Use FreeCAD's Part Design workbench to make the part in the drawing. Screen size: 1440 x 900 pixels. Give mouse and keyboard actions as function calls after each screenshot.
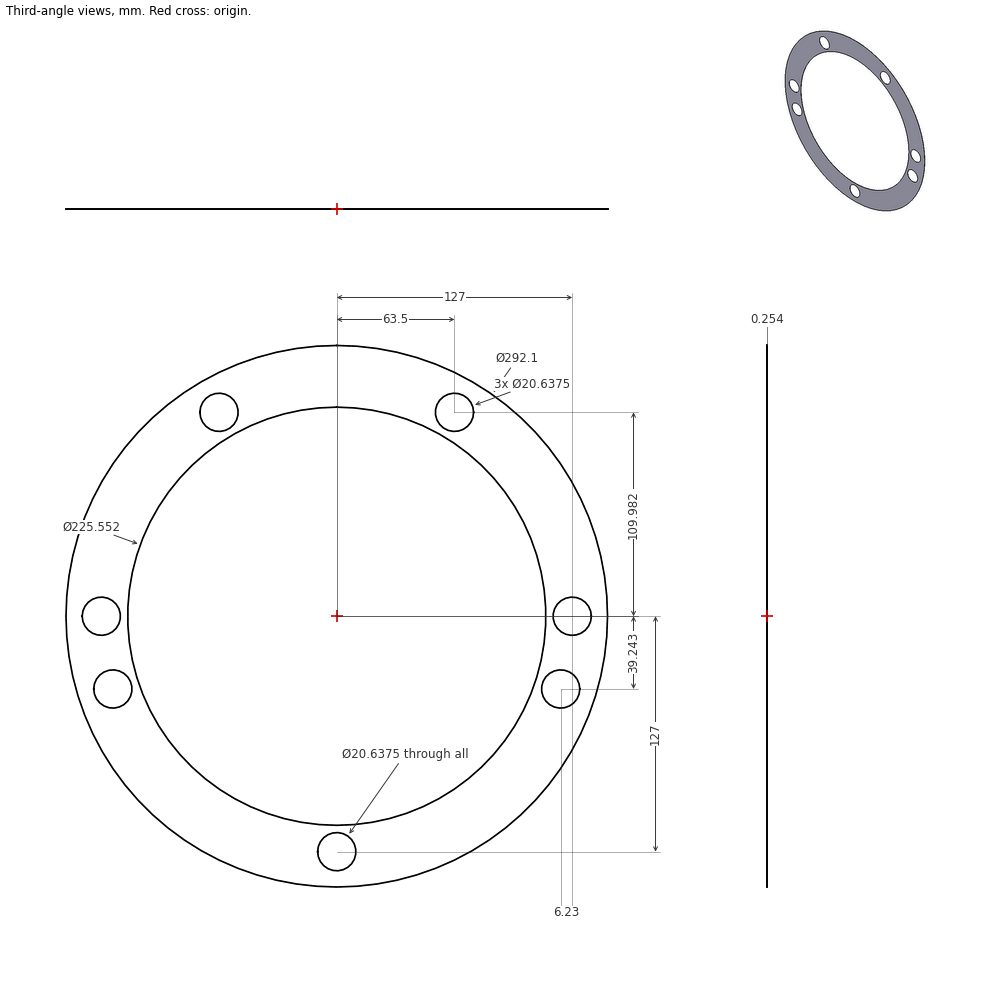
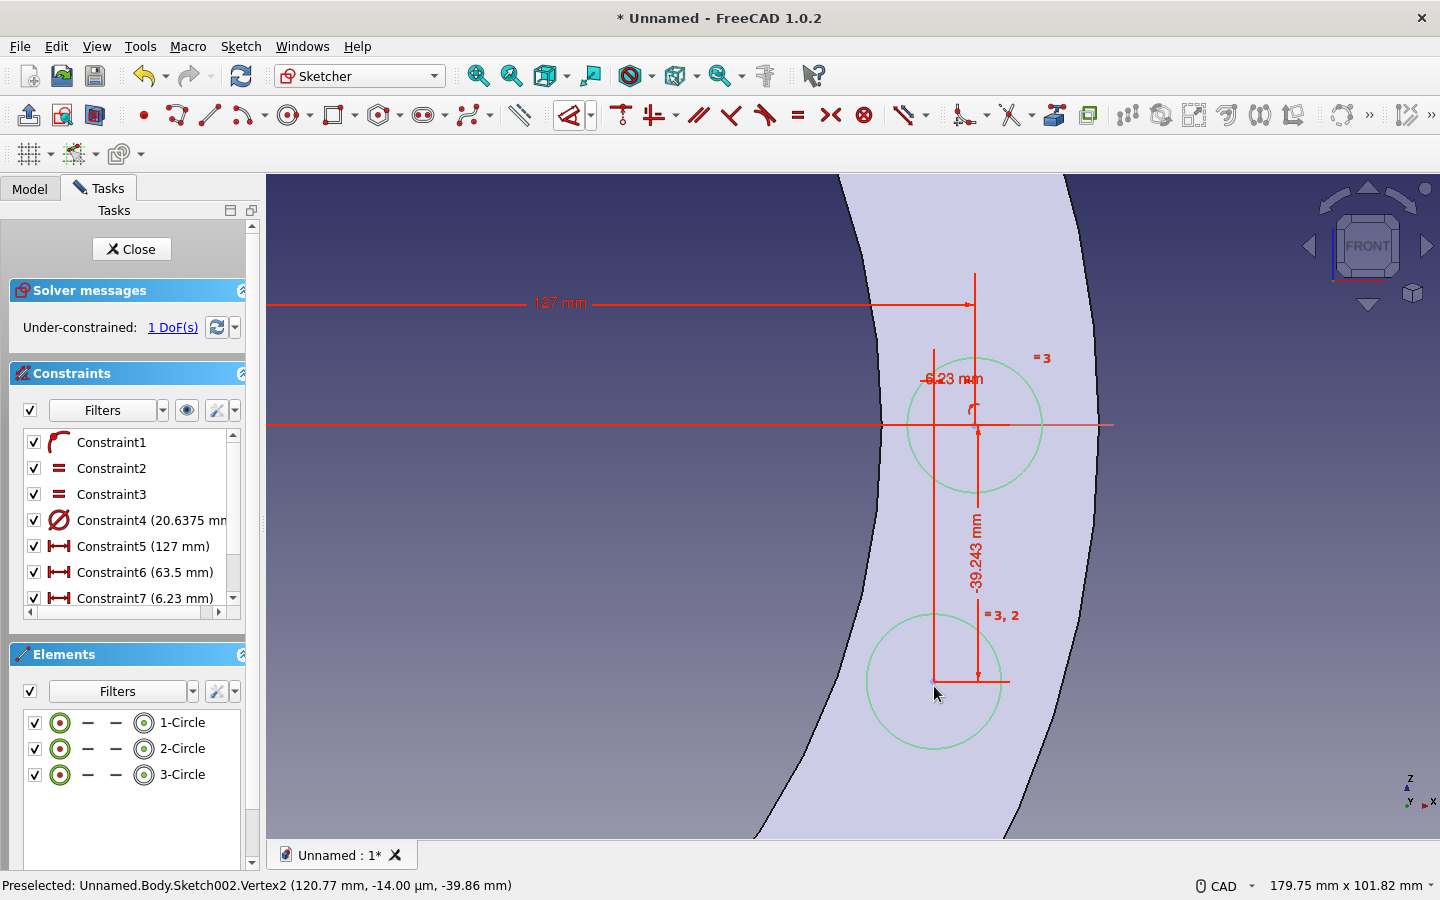
scroll(896, 688, down, 5)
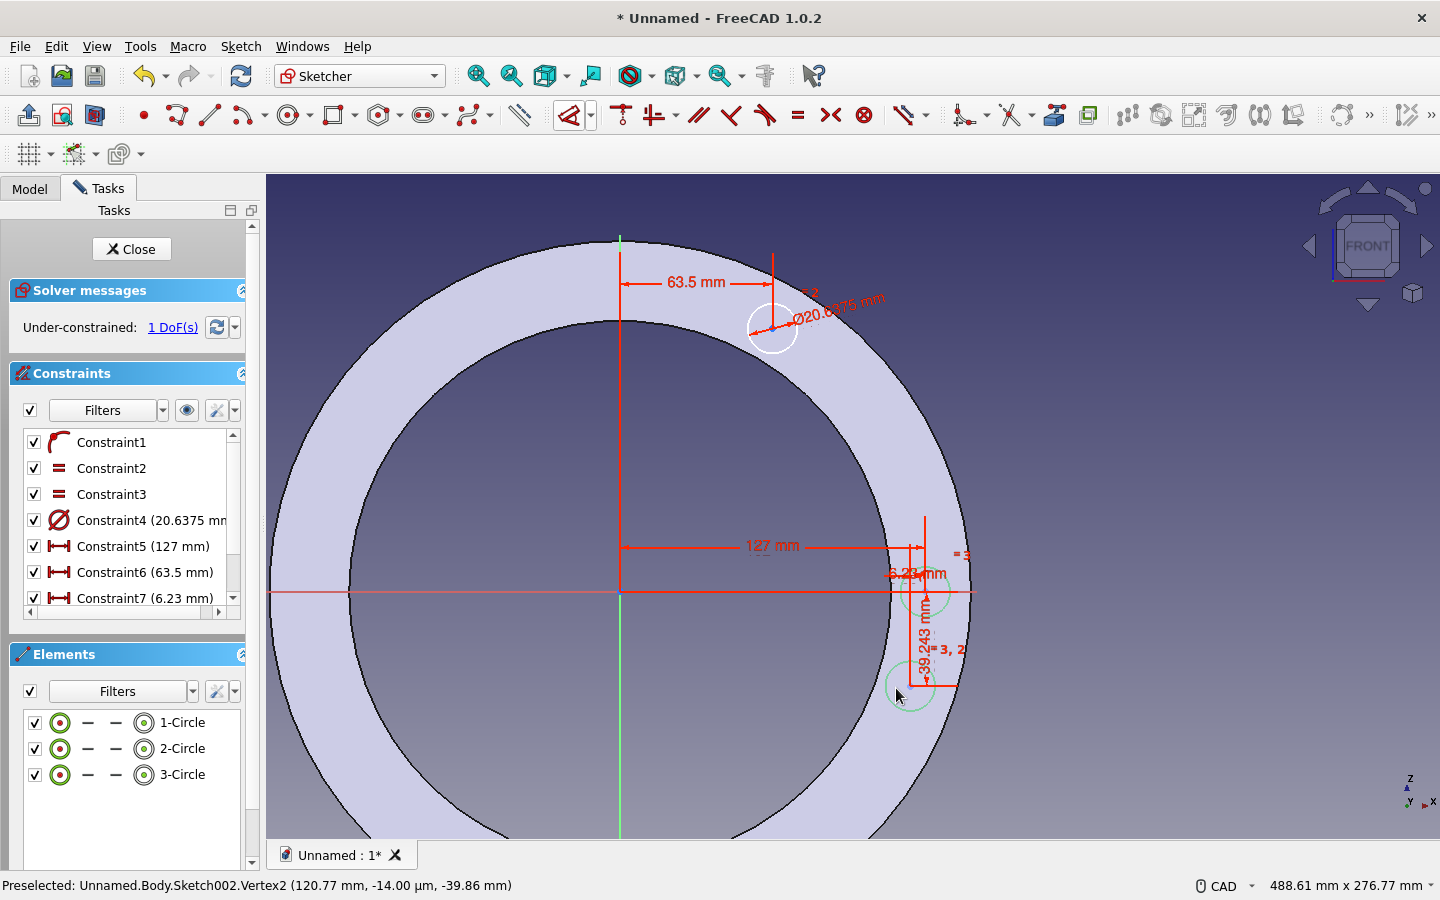
click(773, 329)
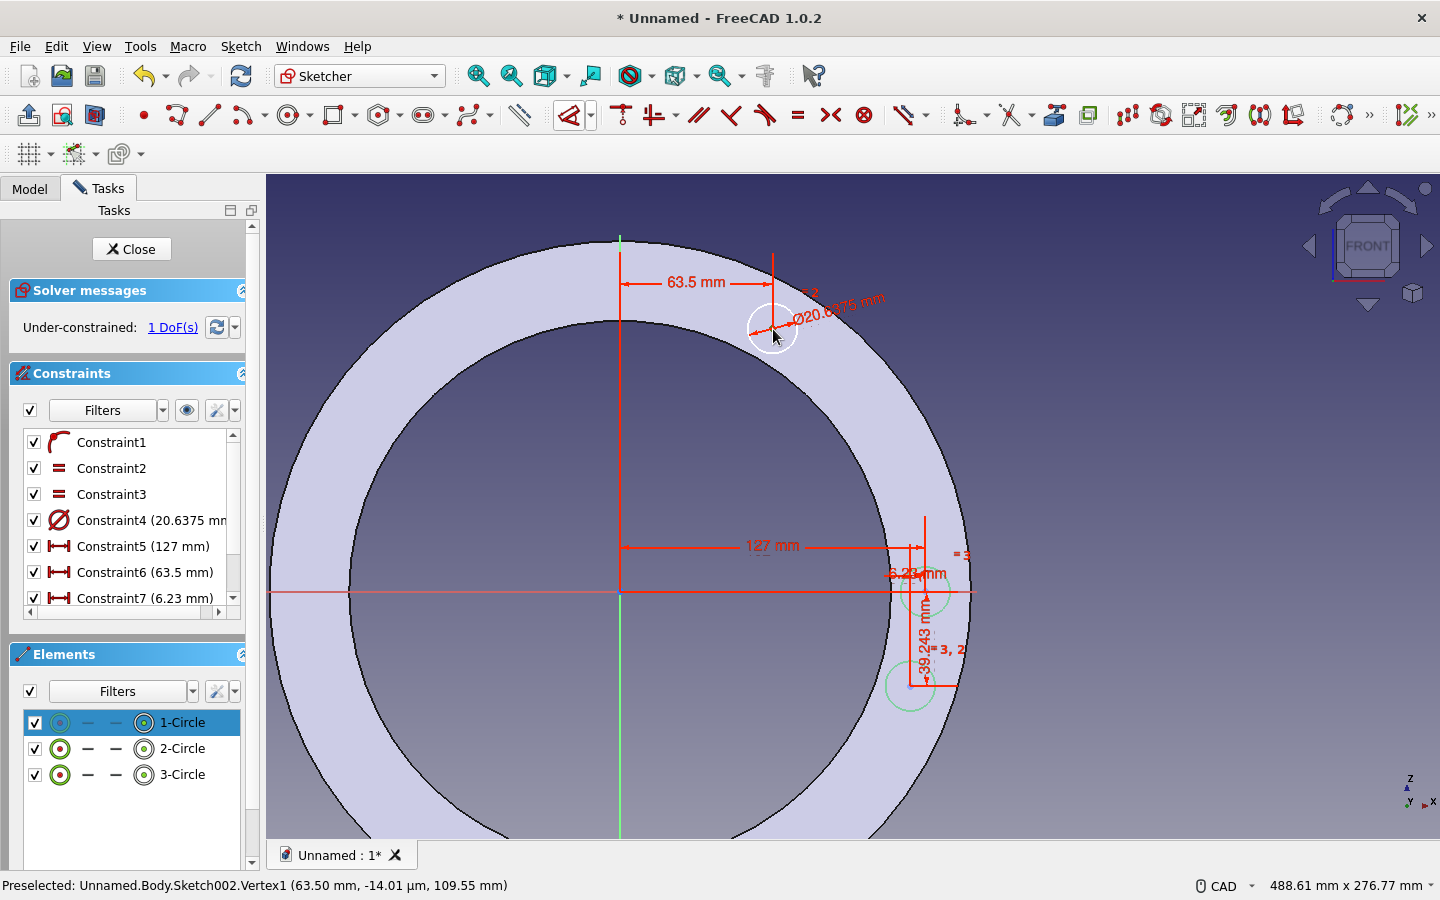
key(i)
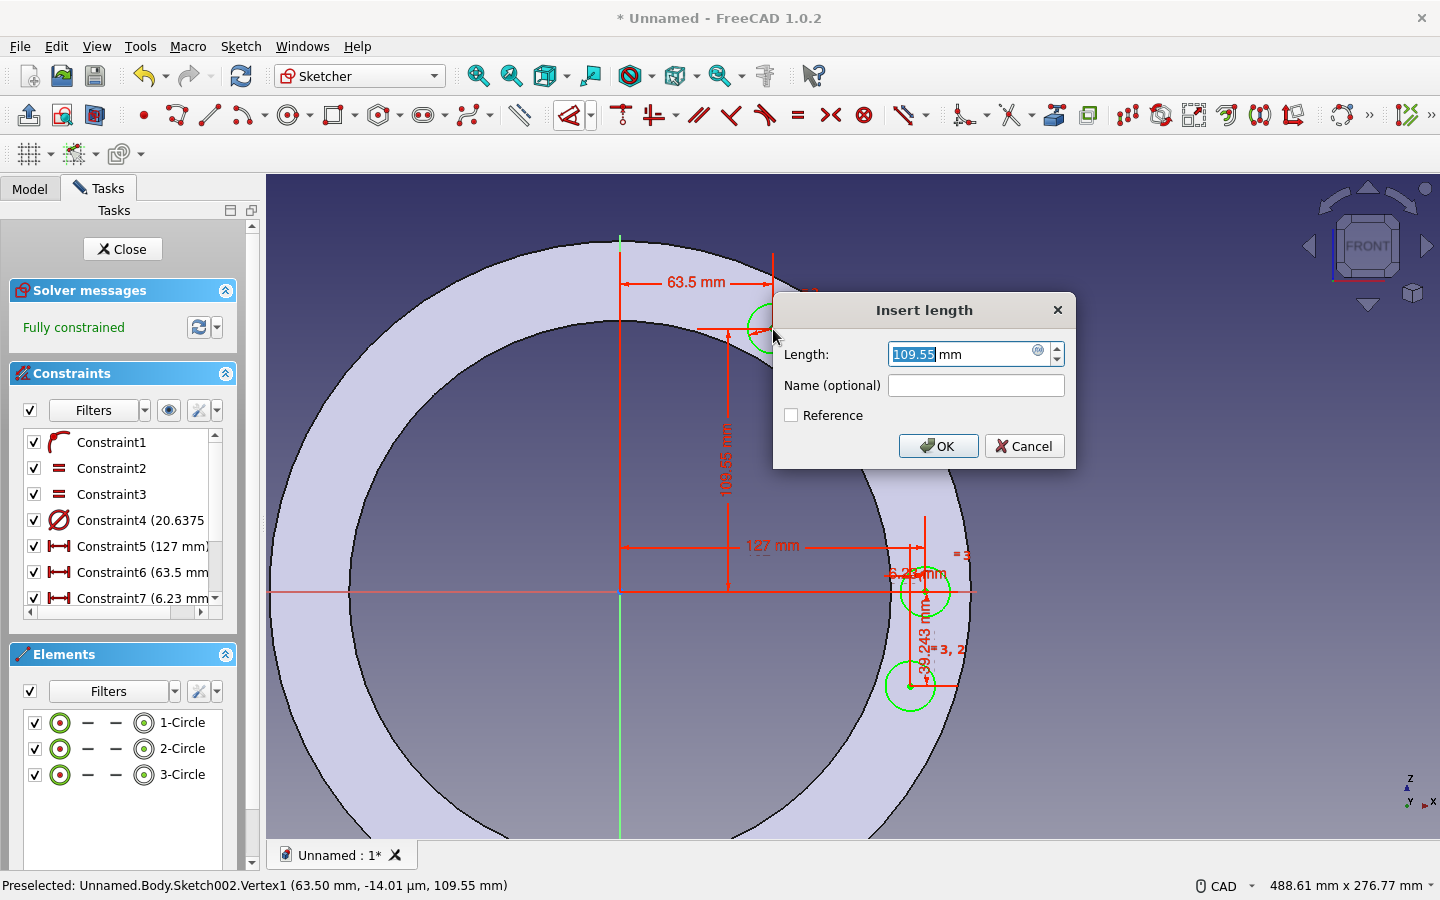
text(109.982)
key(Return)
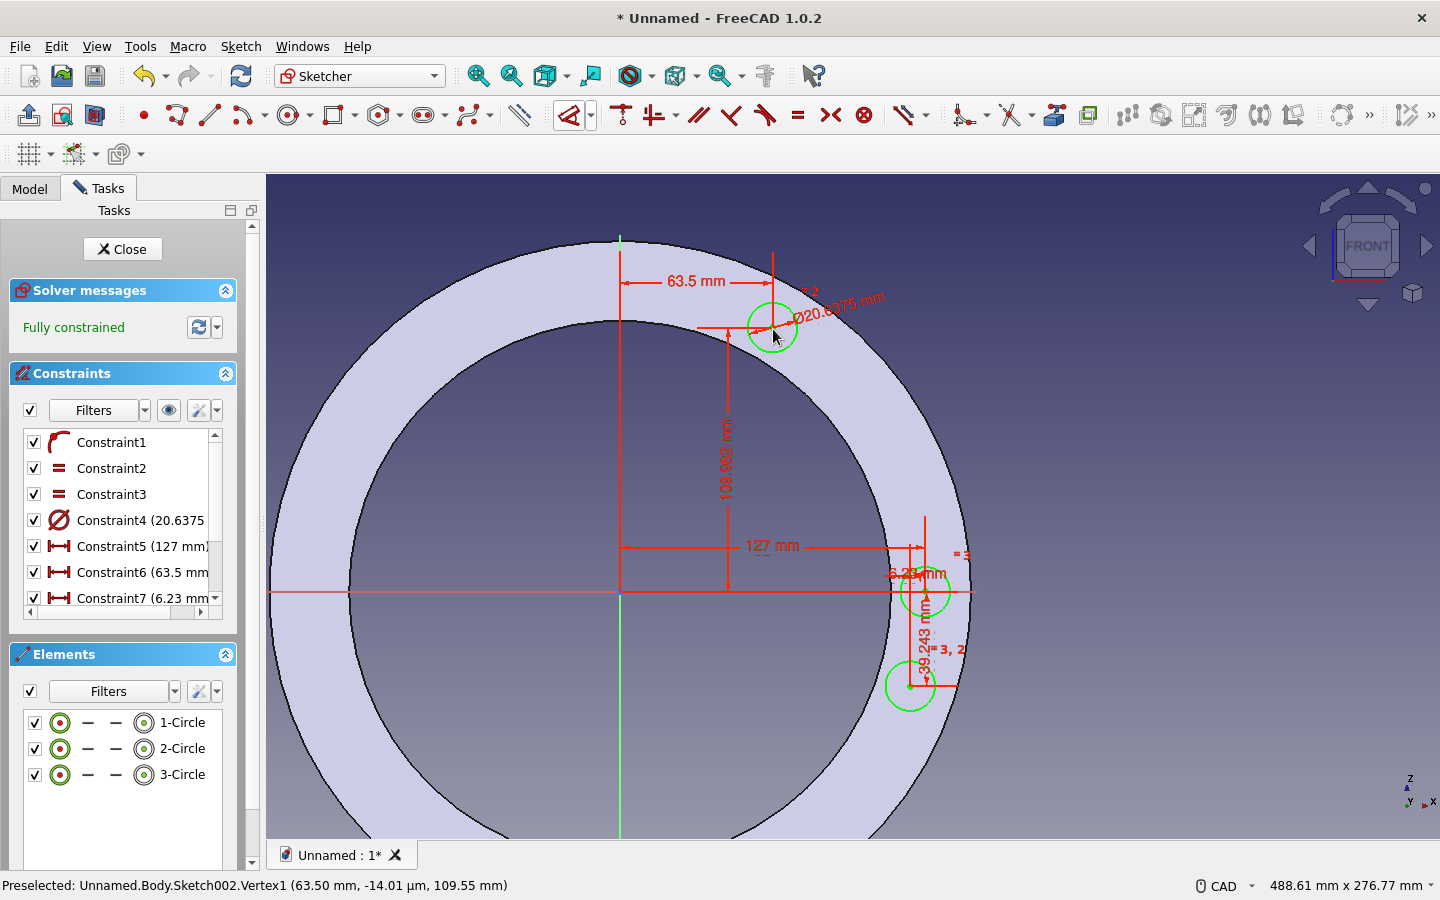
click(123, 249)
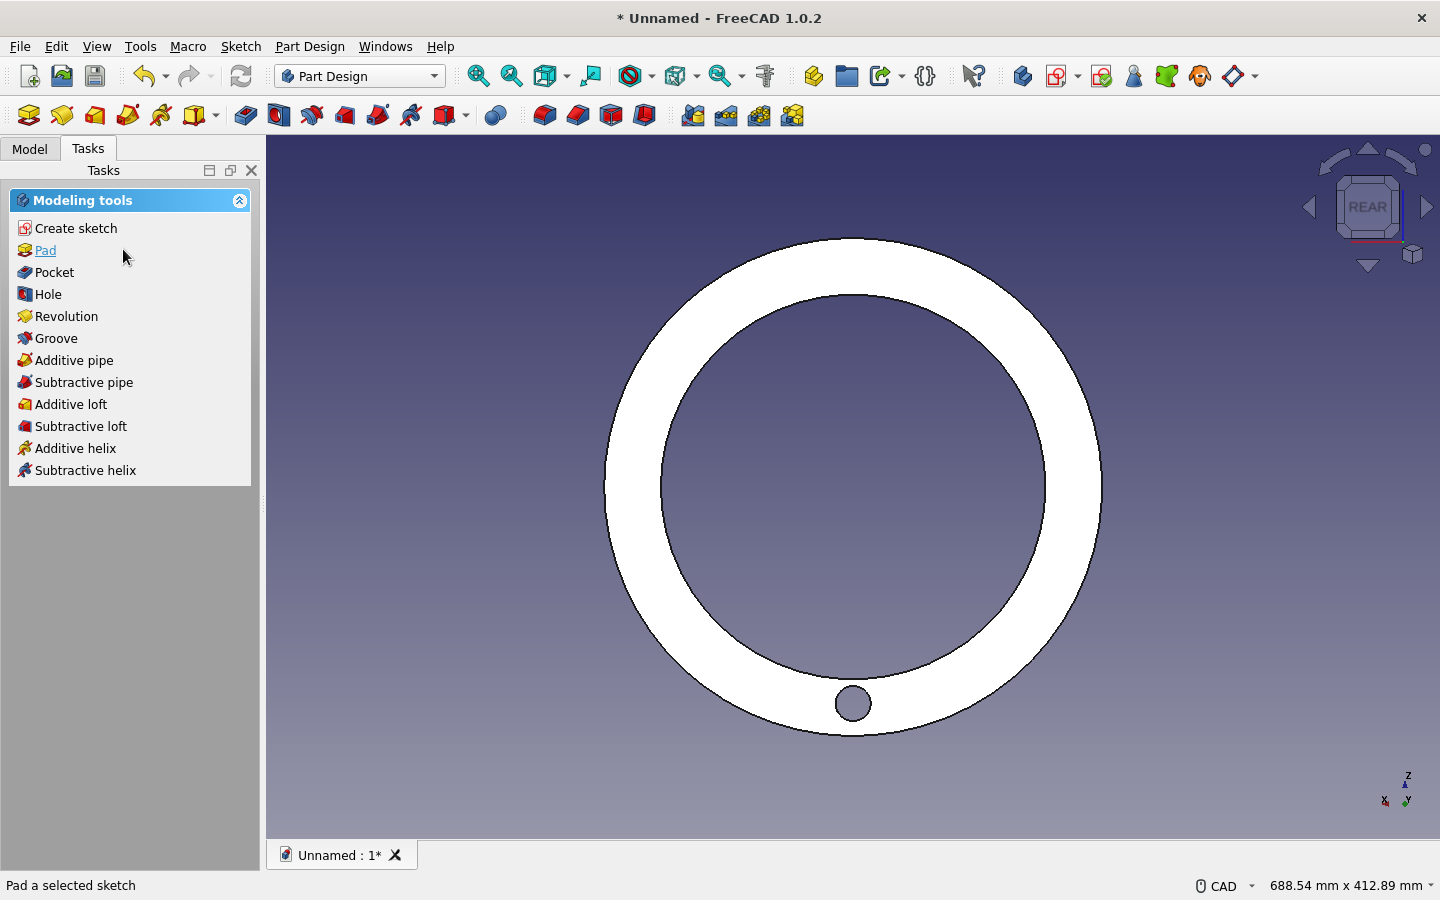
click(246, 116)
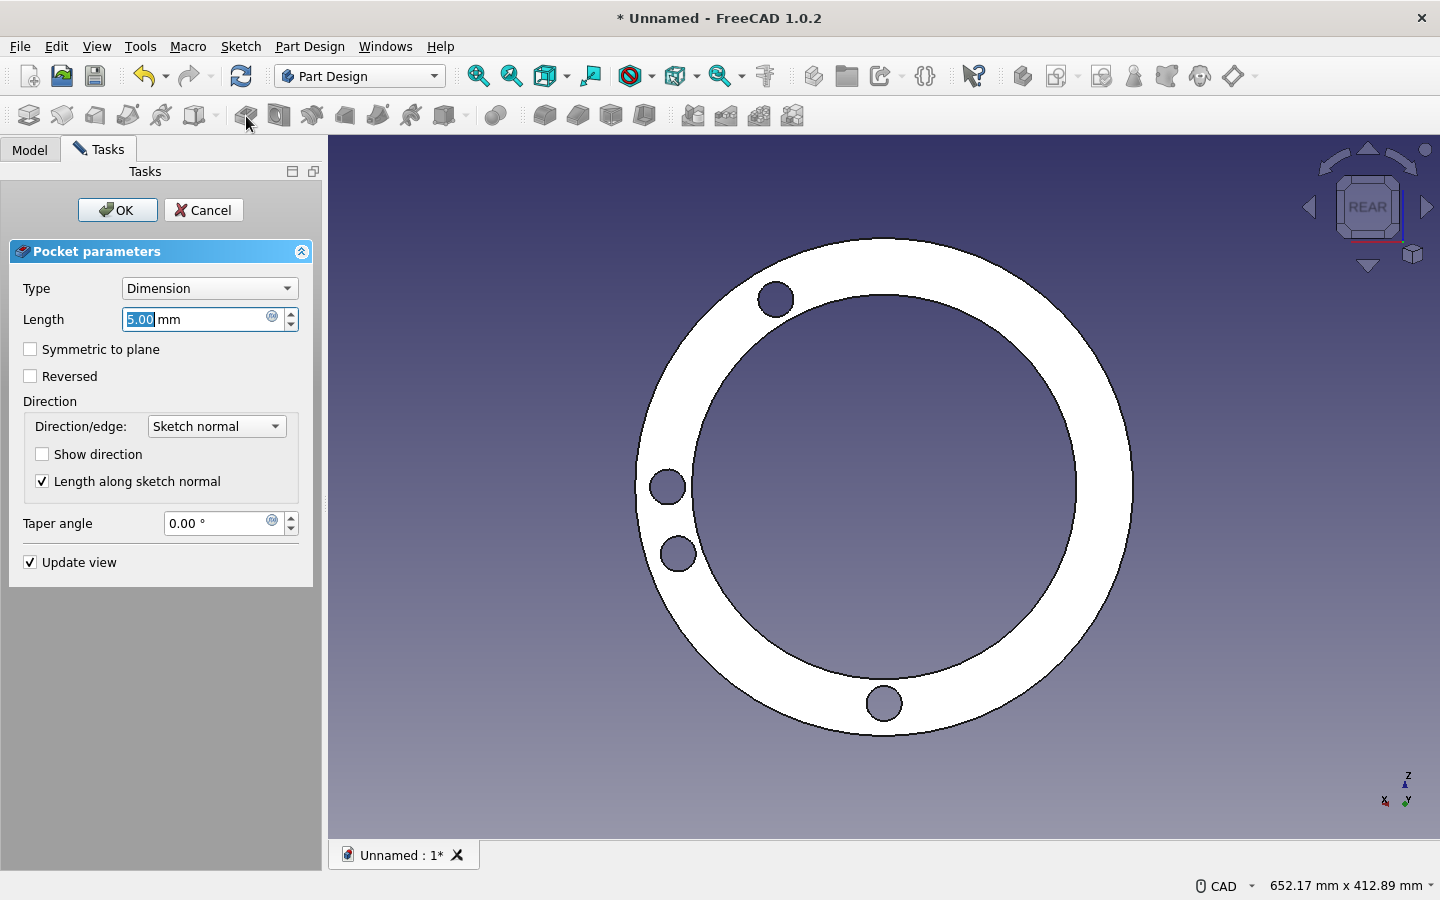
click(210, 288)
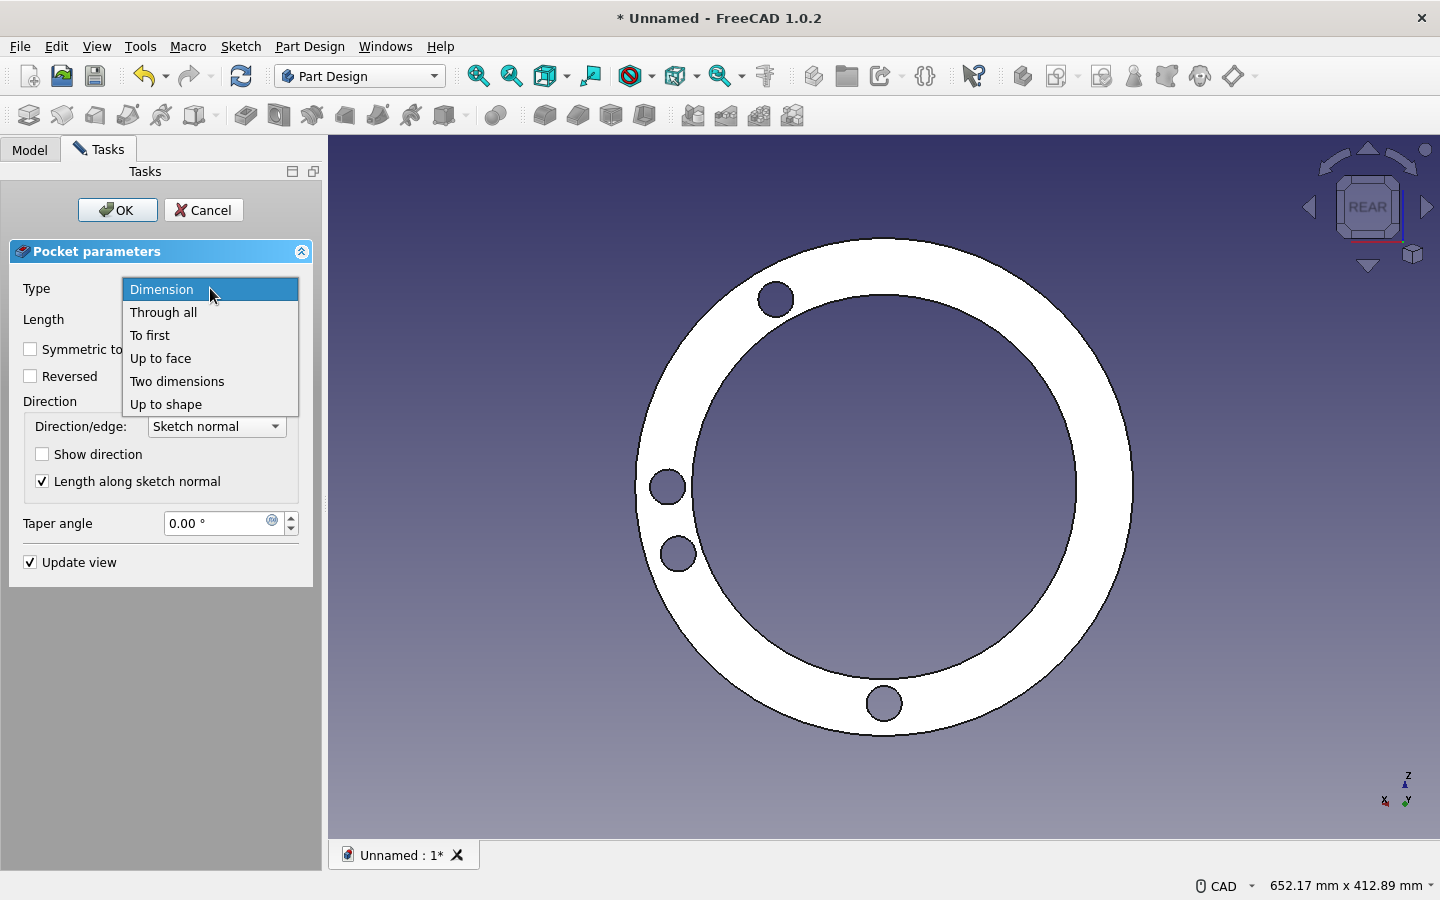
click(208, 312)